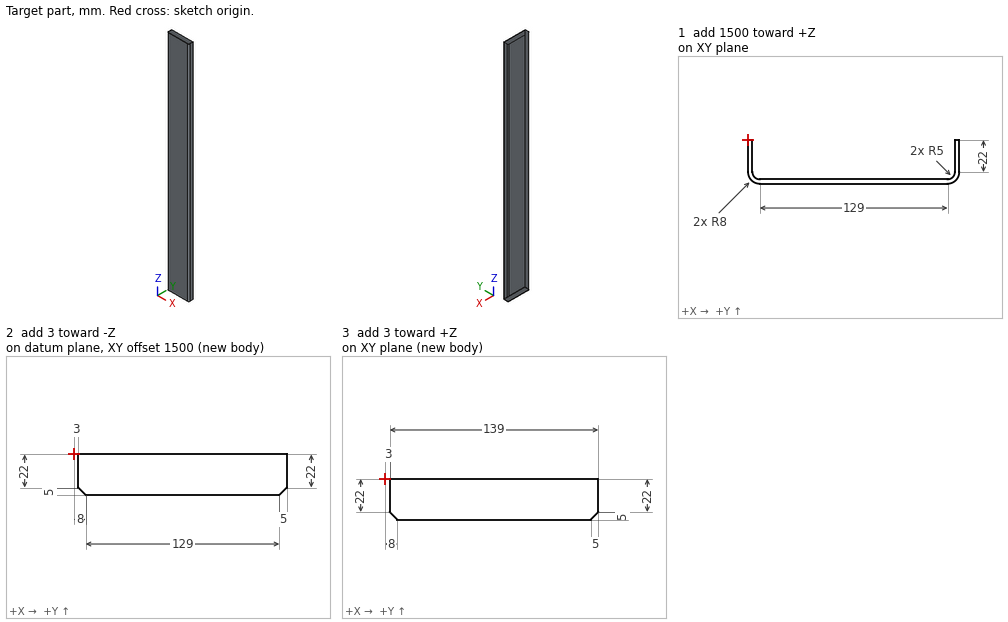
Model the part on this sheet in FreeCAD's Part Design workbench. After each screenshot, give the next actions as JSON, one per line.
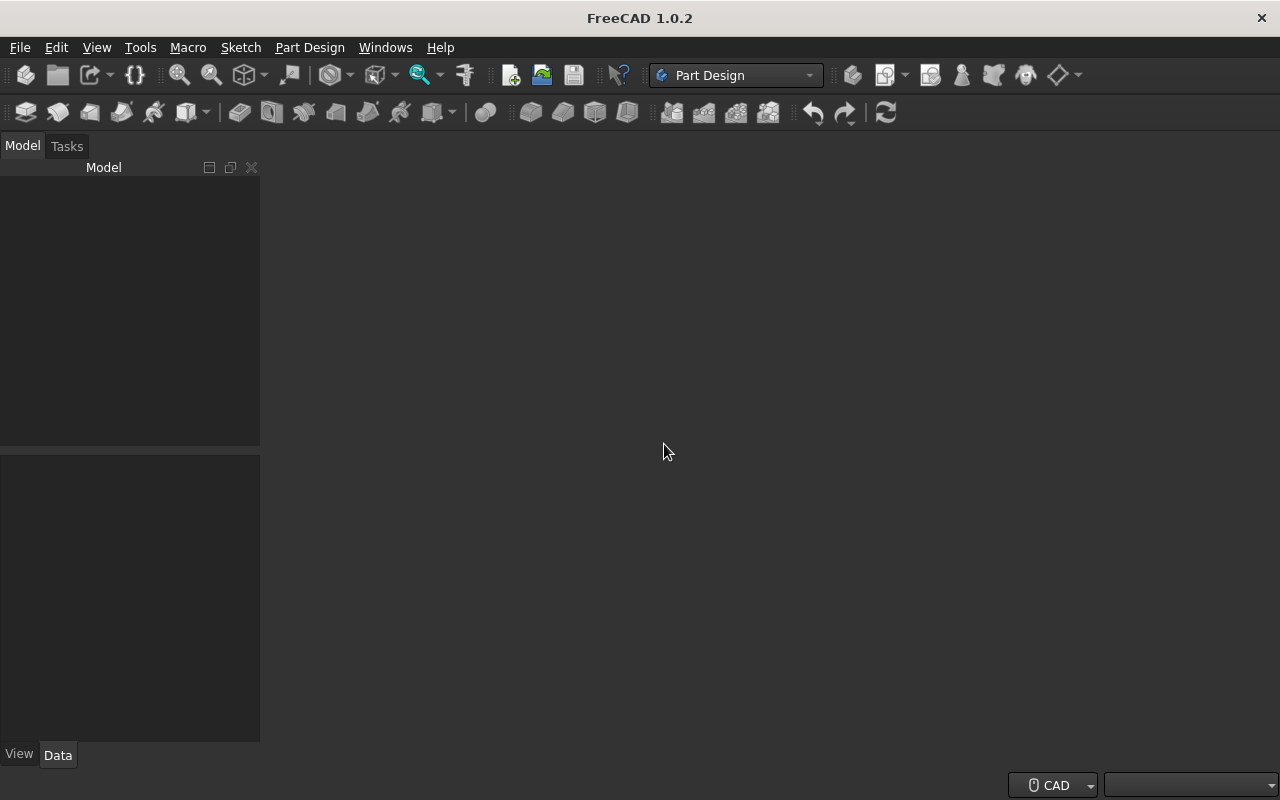
{"action": "key", "text": "ctrl+n"}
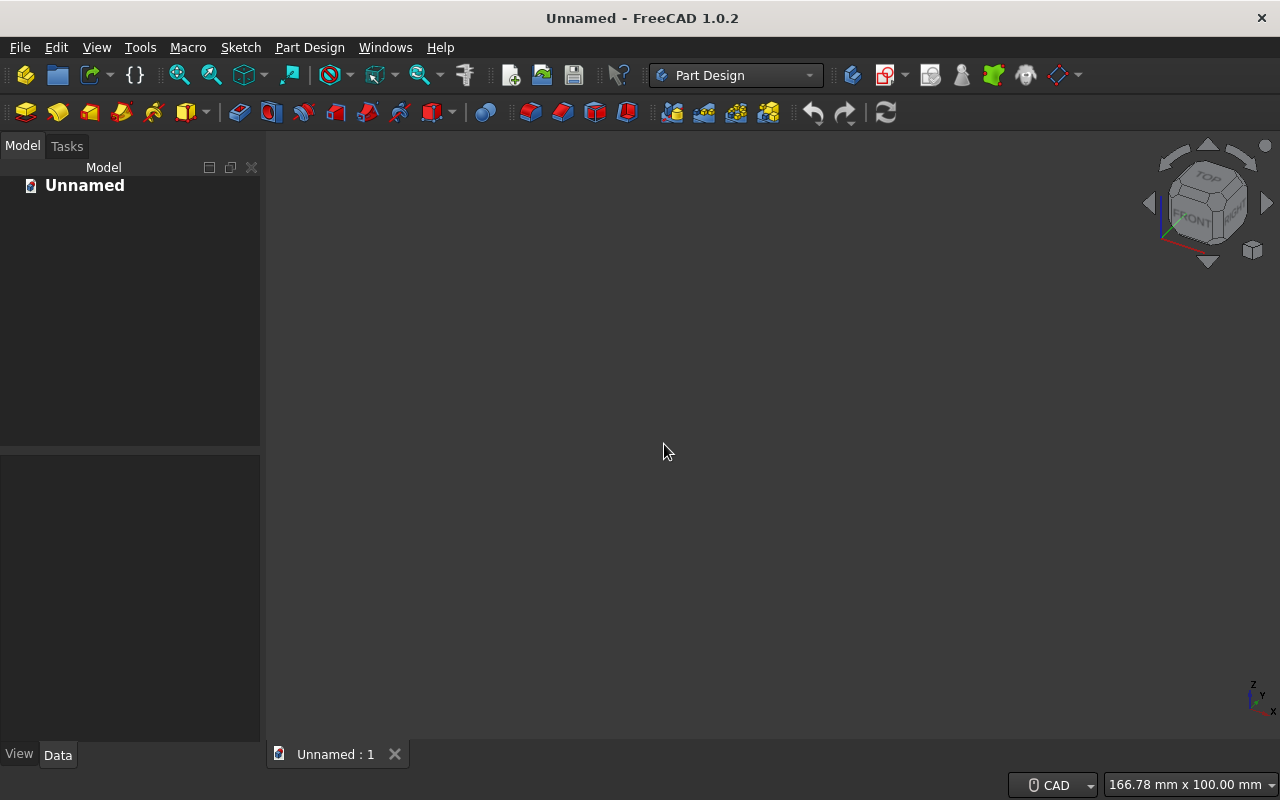
{"action": "left_click", "coordinate": [886, 76]}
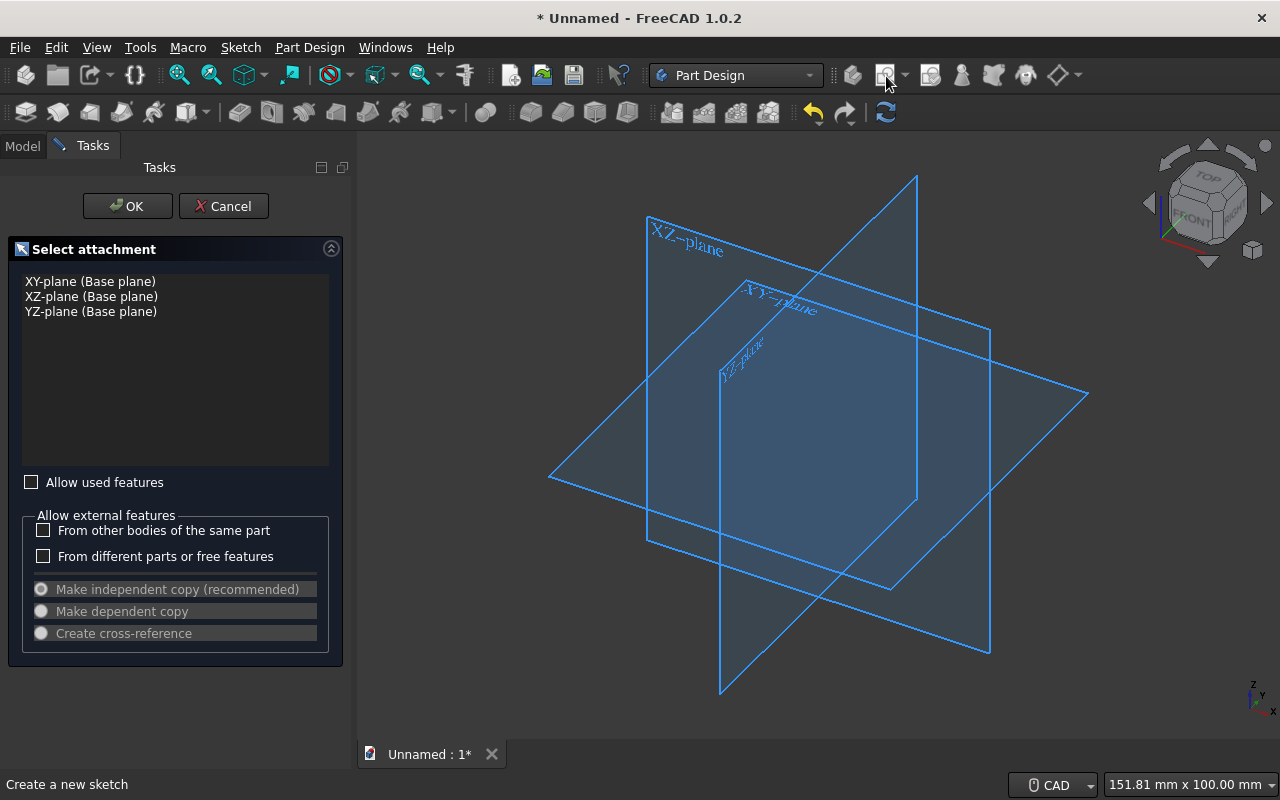
{"action": "left_click", "coordinate": [82, 282]}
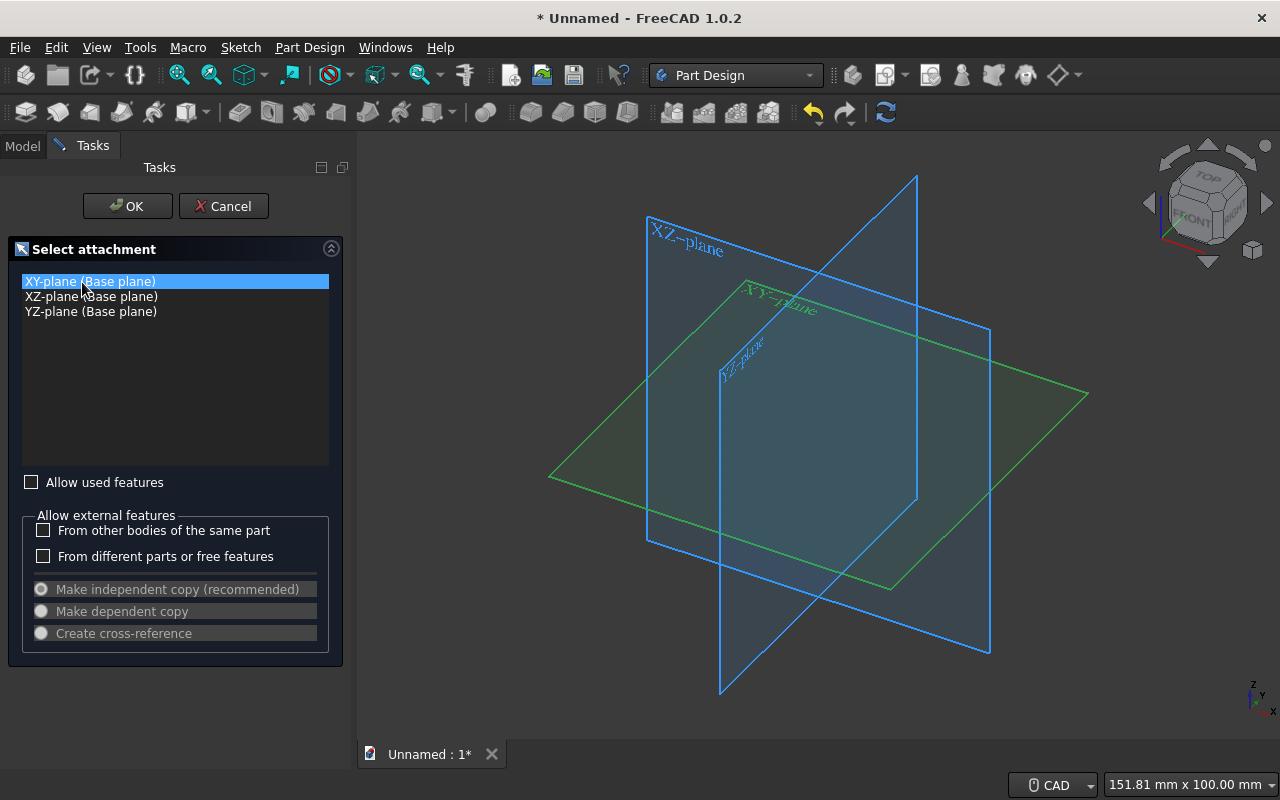
{"action": "left_click", "coordinate": [128, 206]}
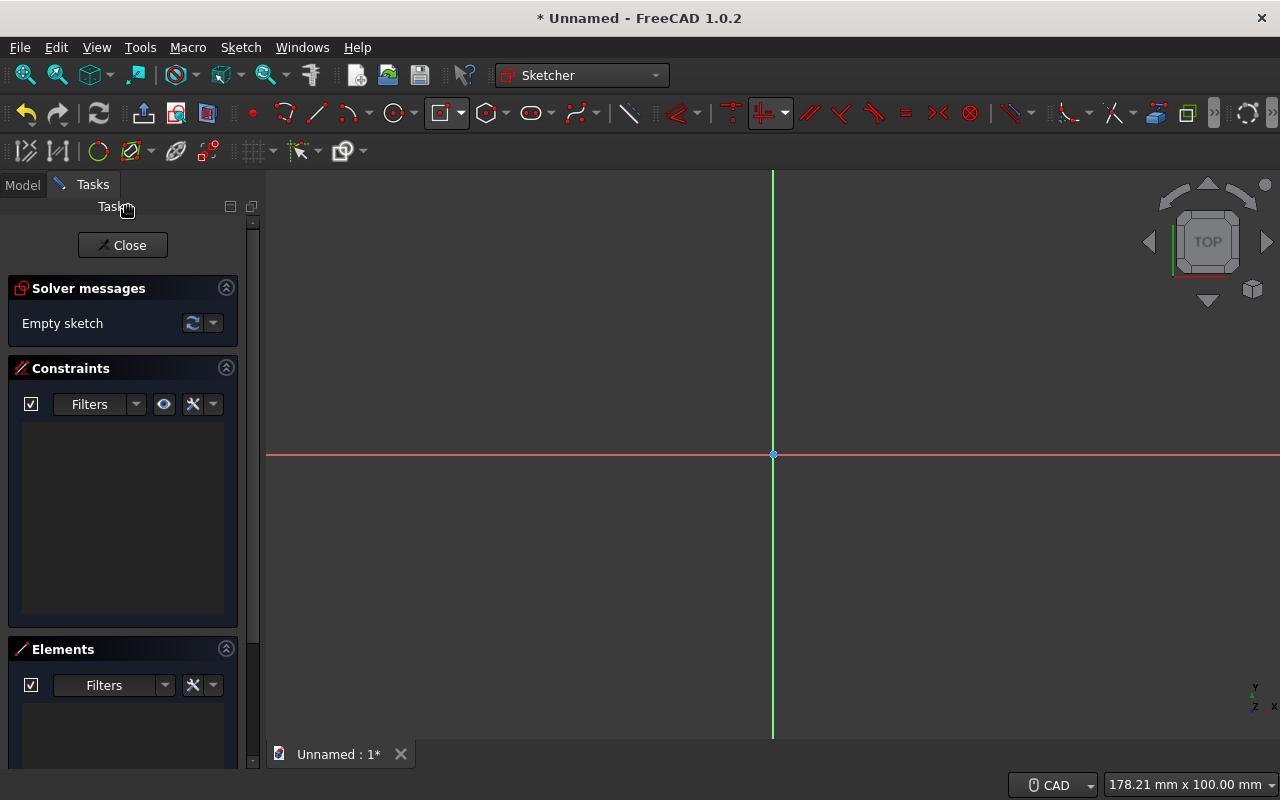
{"action": "scroll", "coordinate": [294, 351], "scroll_direction": "down", "scroll_amount": 3}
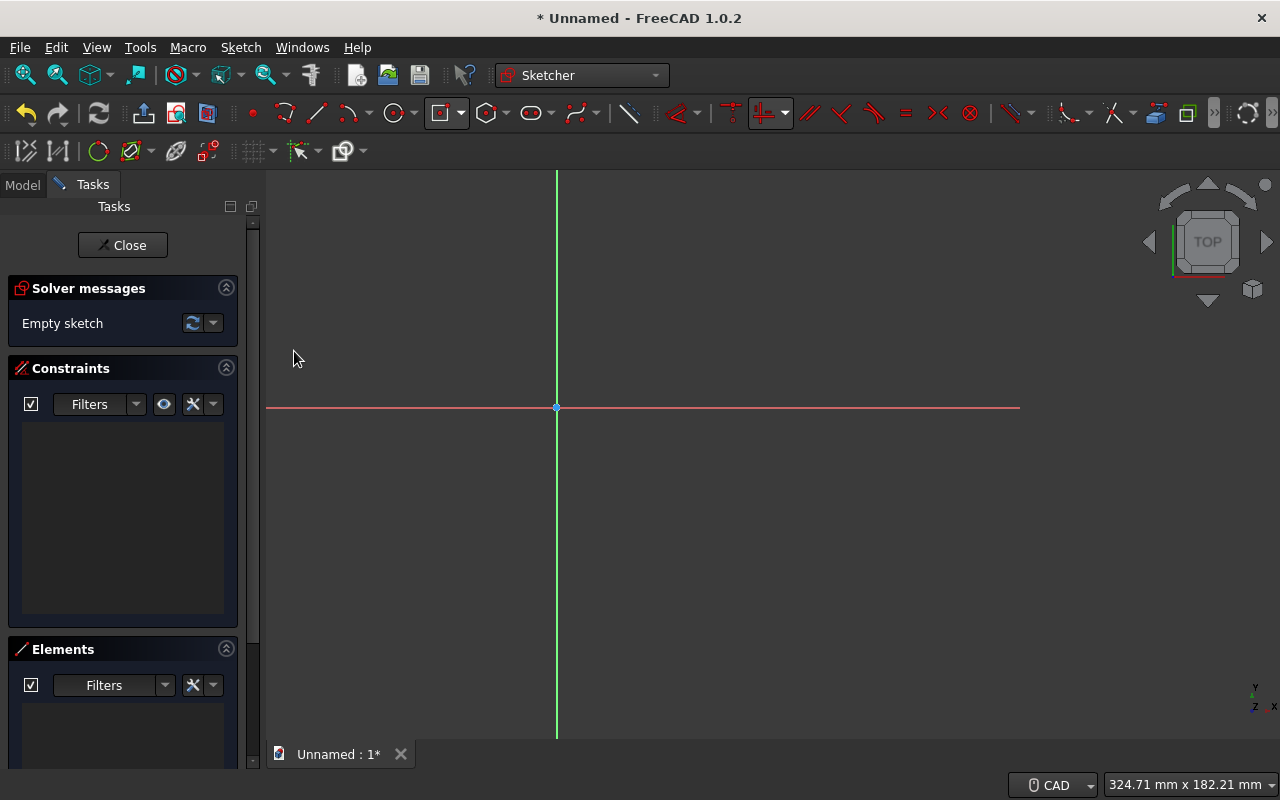
{"action": "key", "text": "g l"}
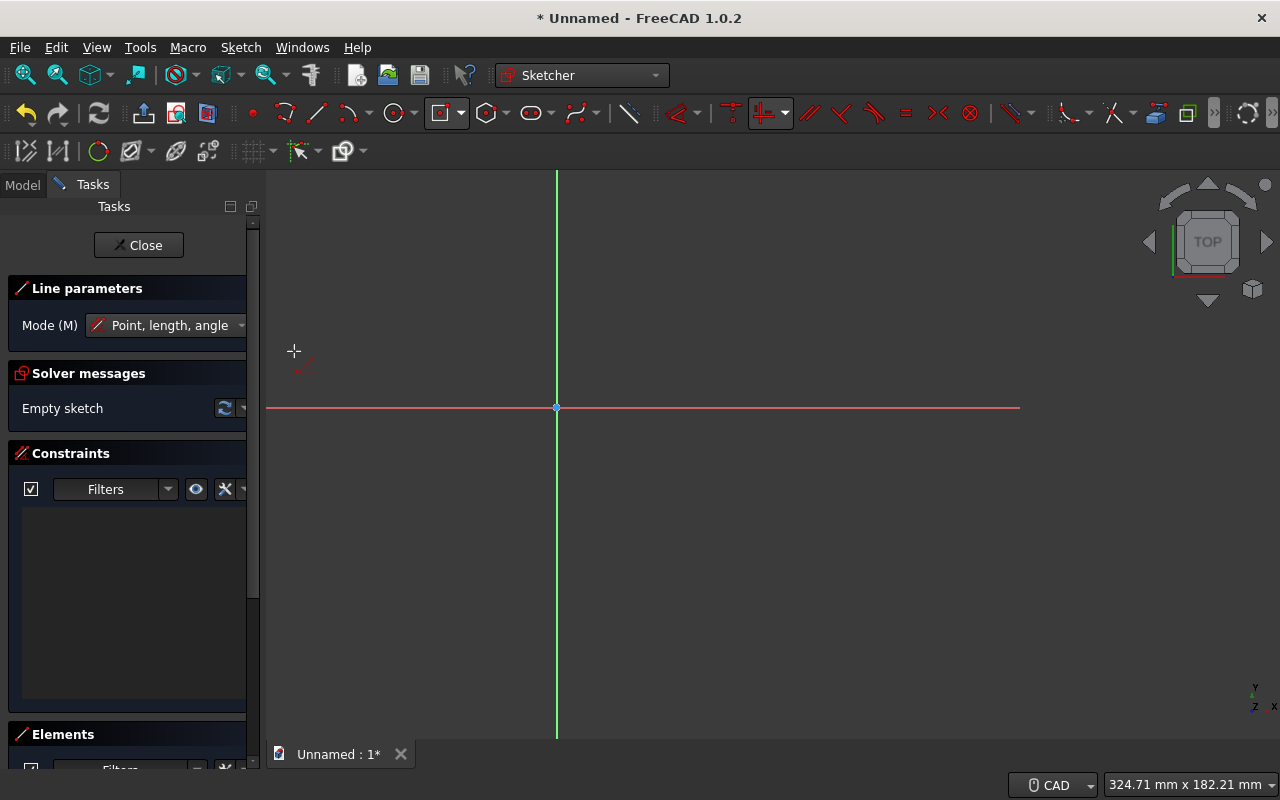
{"action": "left_click", "coordinate": [582, 502]}
{"action": "left_click", "coordinate": [985, 502]}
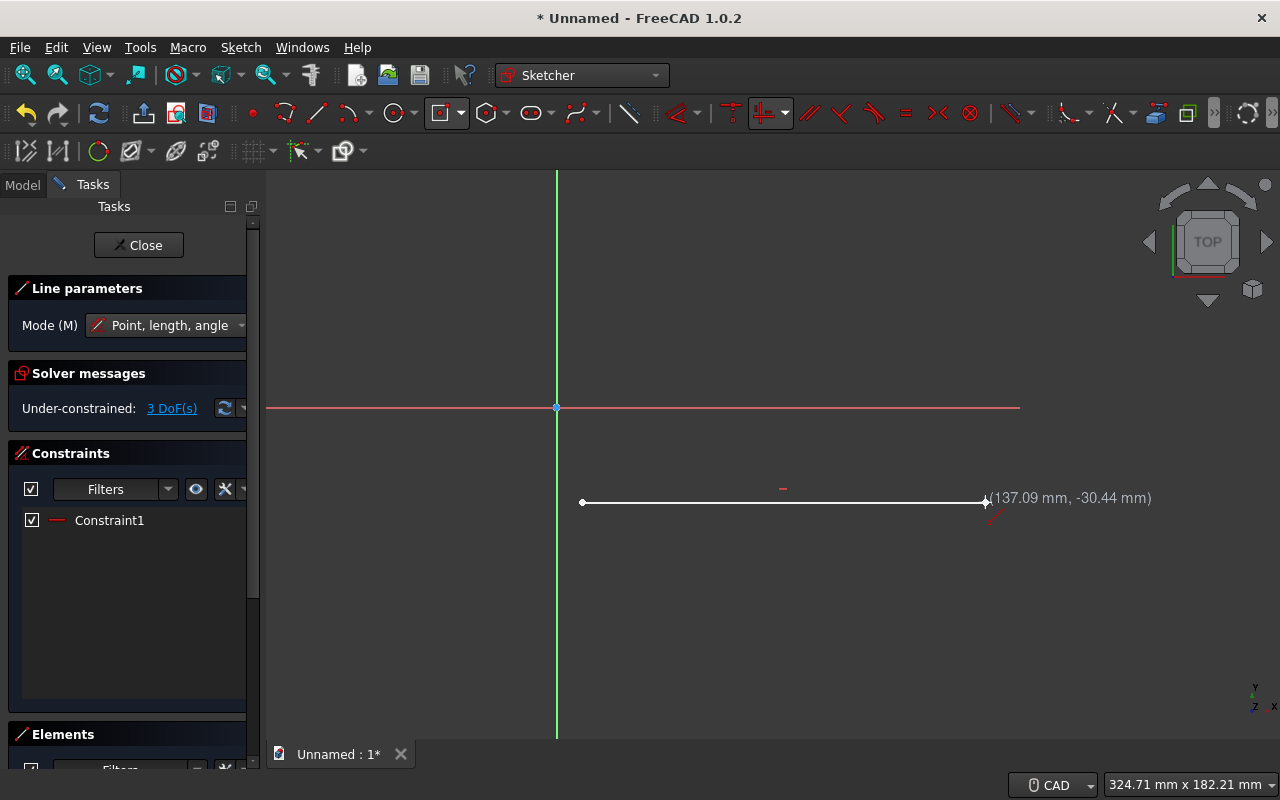
{"action": "left_click", "coordinate": [286, 114]}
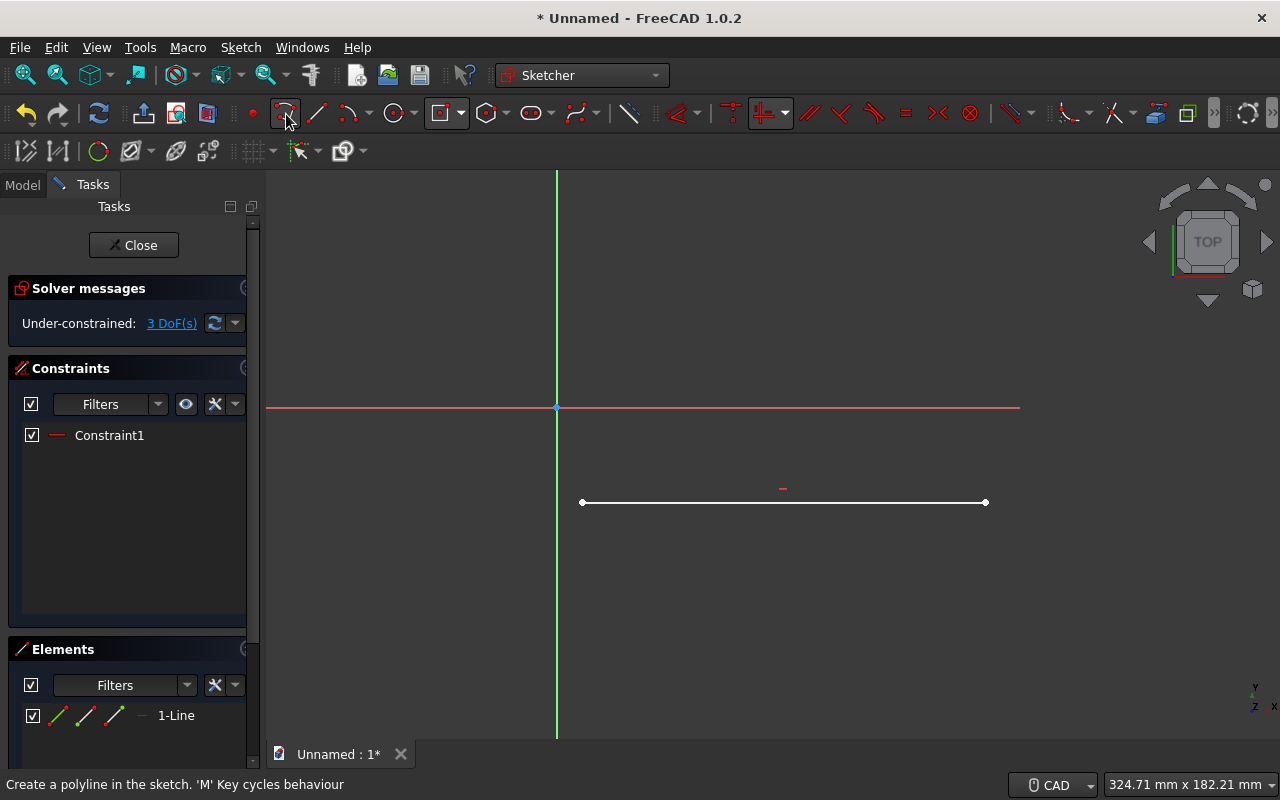
{"action": "left_click", "coordinate": [1010, 477]}
{"action": "left_click", "coordinate": [1010, 408]}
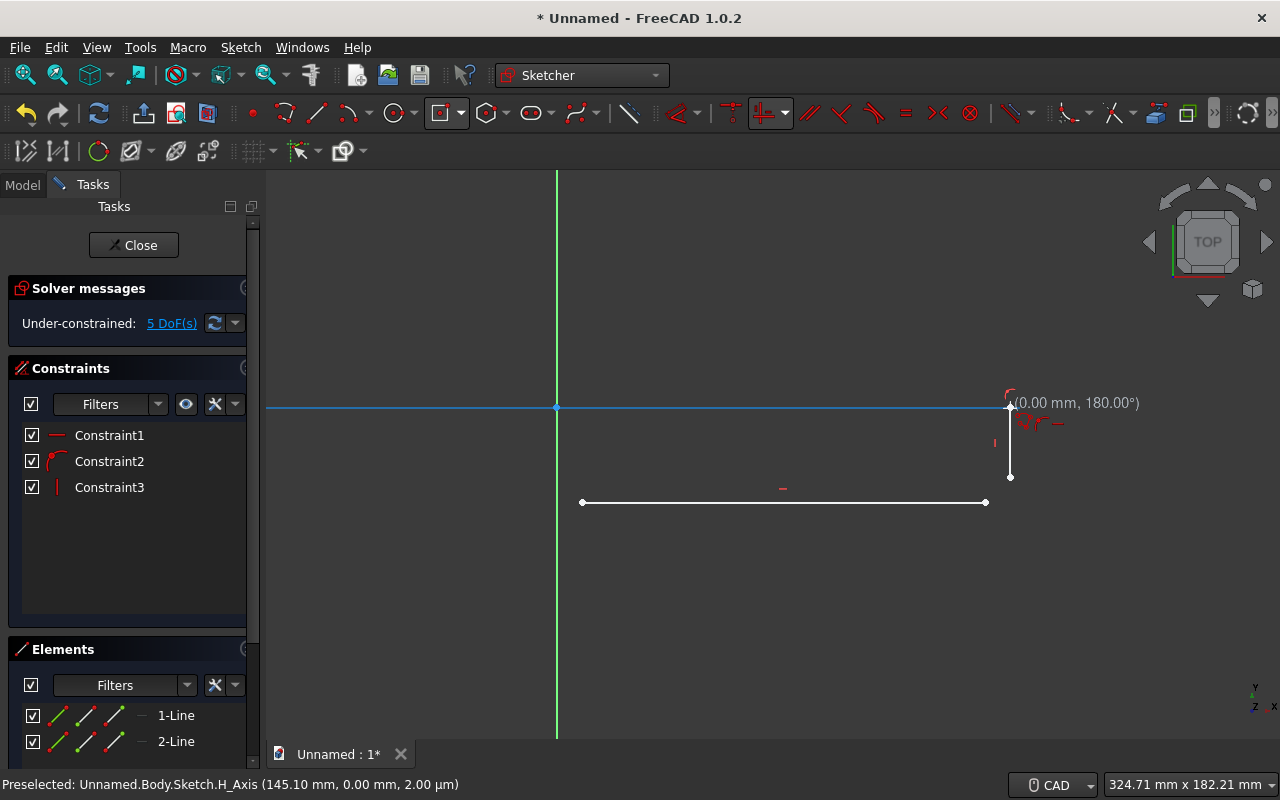
{"action": "scroll", "coordinate": [1000, 408], "scroll_direction": "up", "scroll_amount": 3}